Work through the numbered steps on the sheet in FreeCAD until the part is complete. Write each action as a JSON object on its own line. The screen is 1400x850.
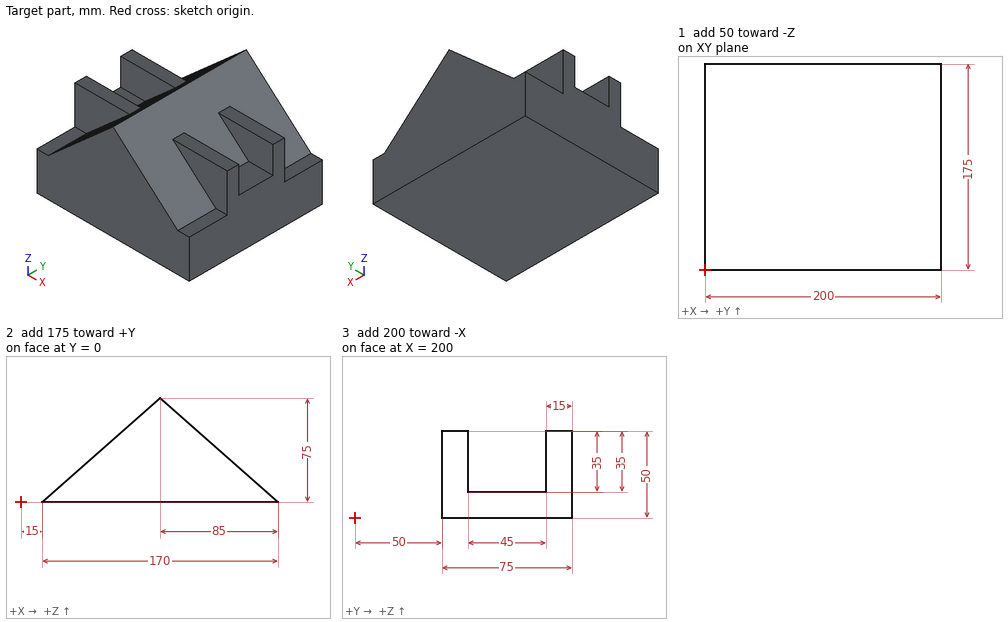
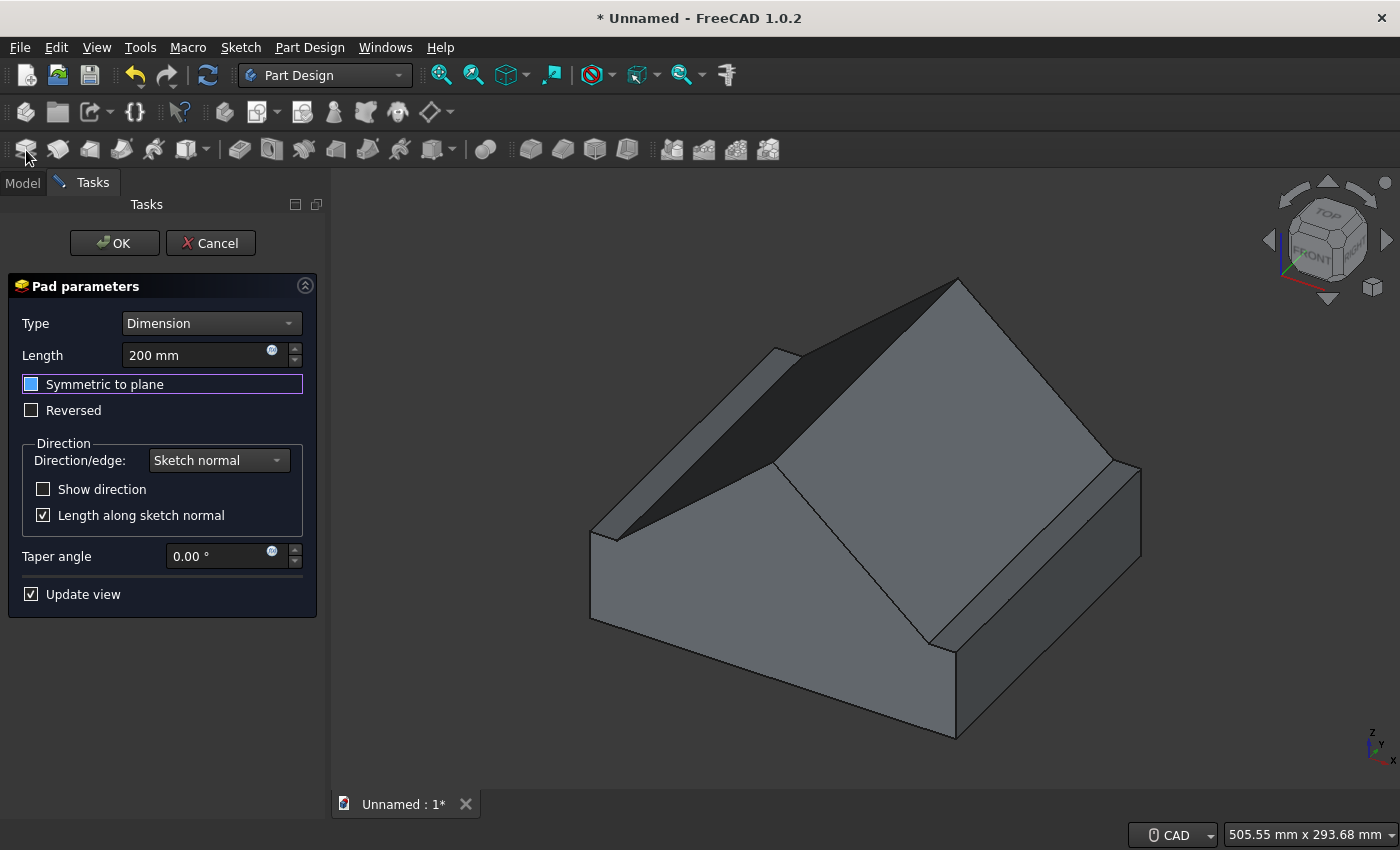
{"action": "left_click", "coordinate": [30, 410]}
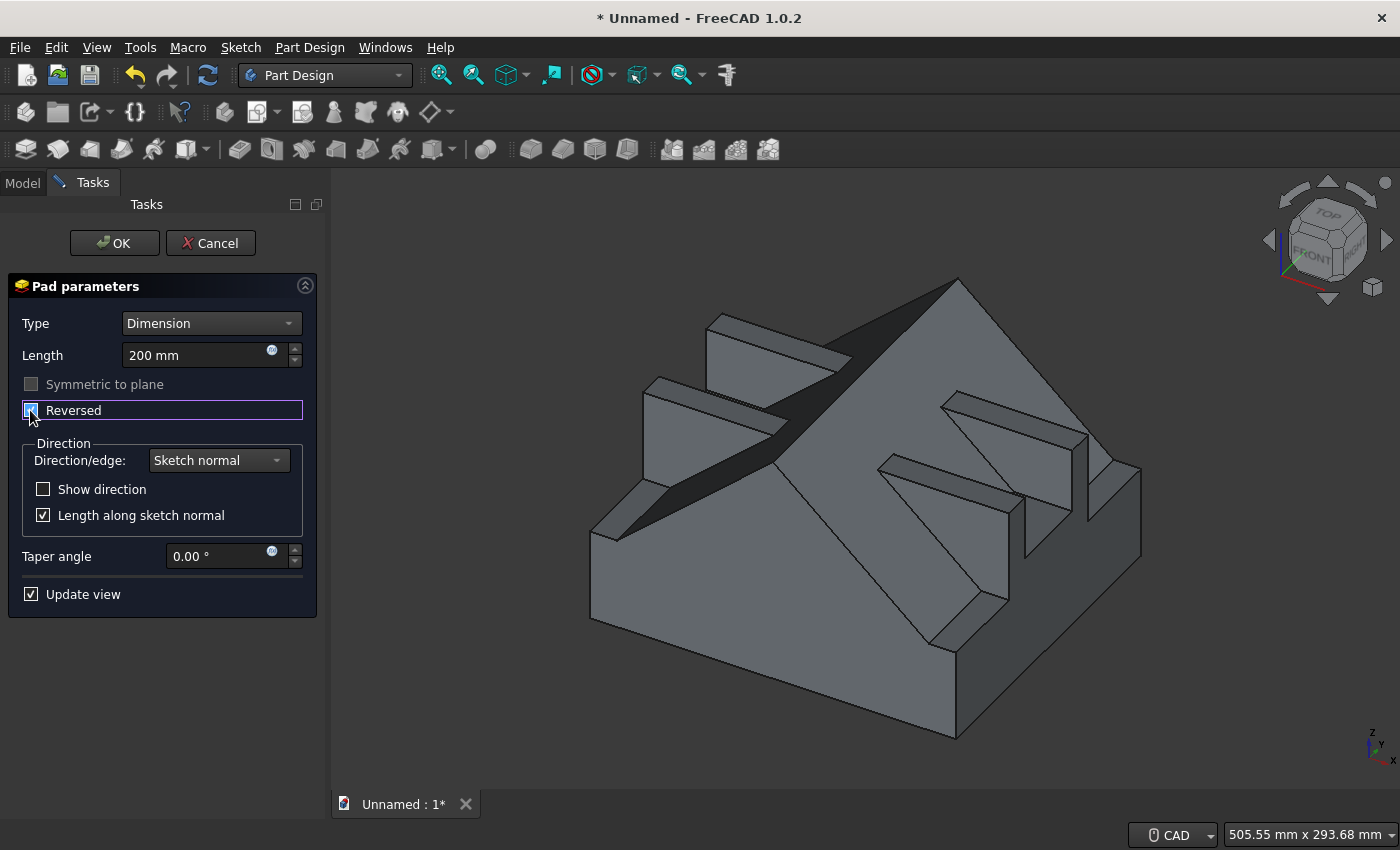
{"action": "left_click", "coordinate": [115, 243]}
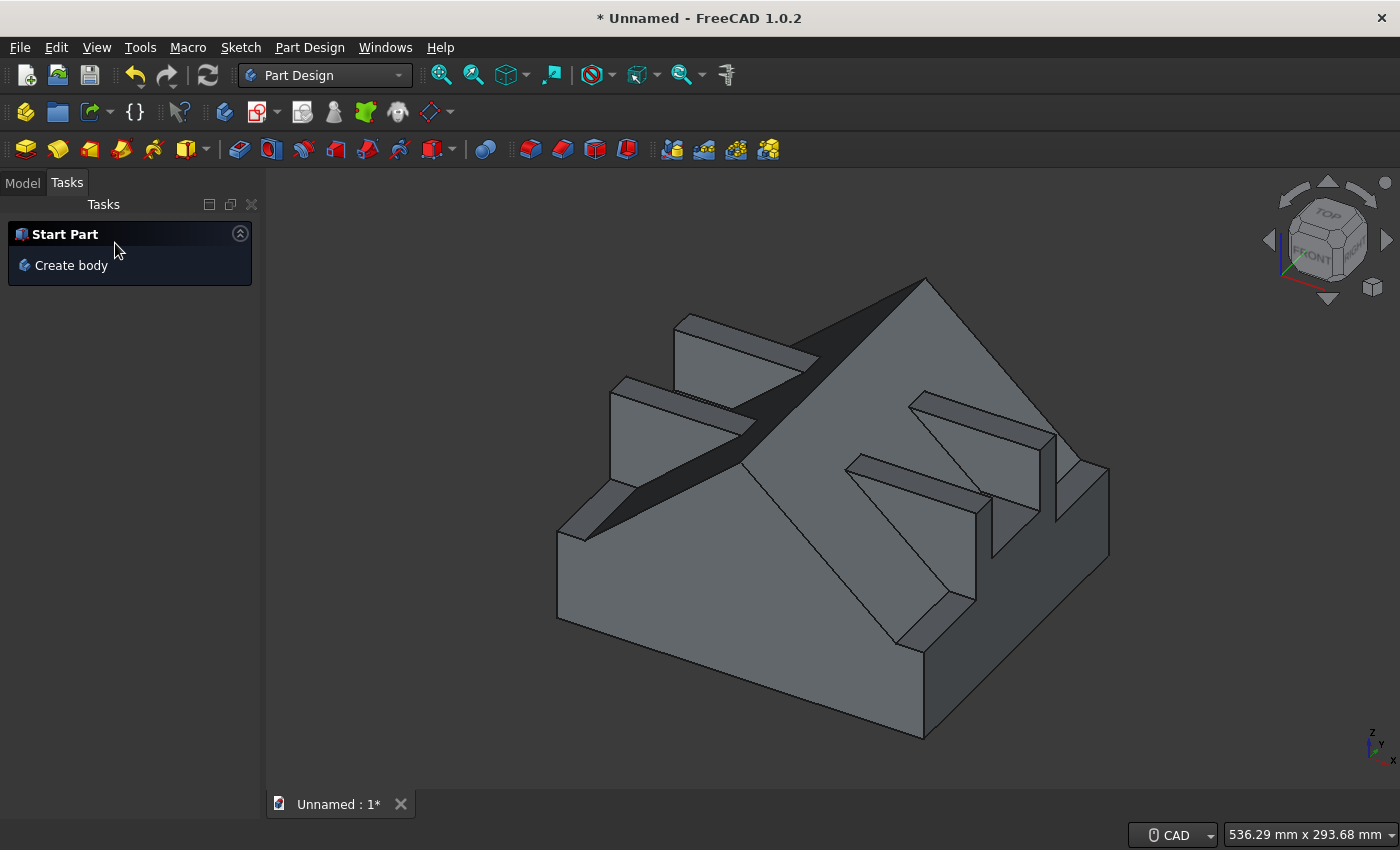
{"action": "key", "text": "0"}